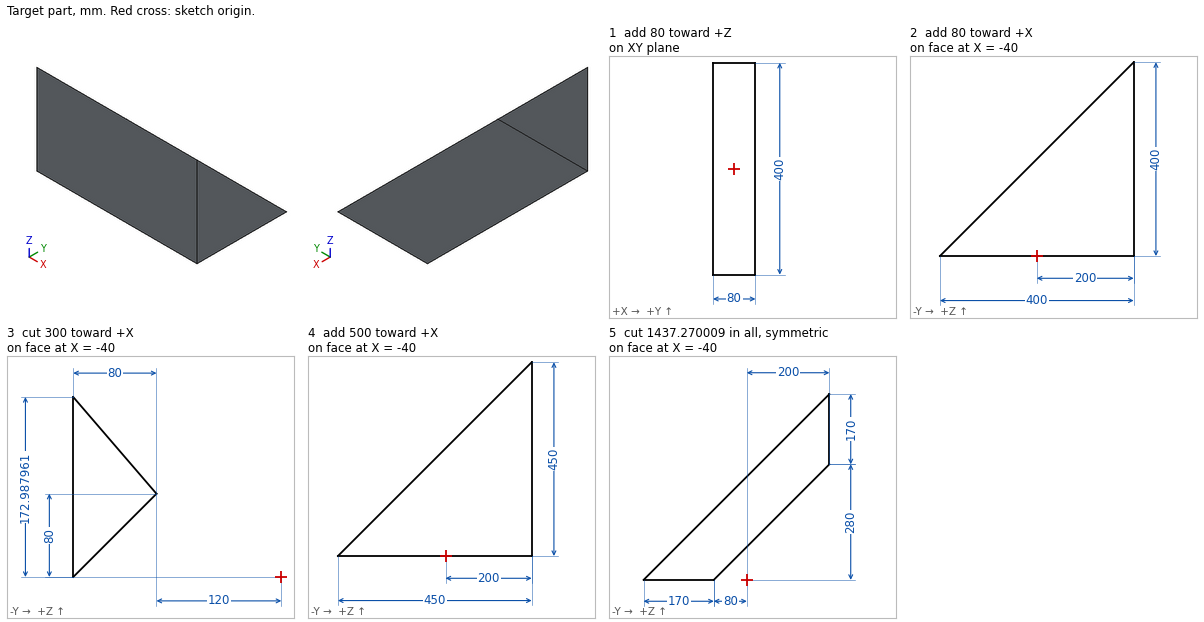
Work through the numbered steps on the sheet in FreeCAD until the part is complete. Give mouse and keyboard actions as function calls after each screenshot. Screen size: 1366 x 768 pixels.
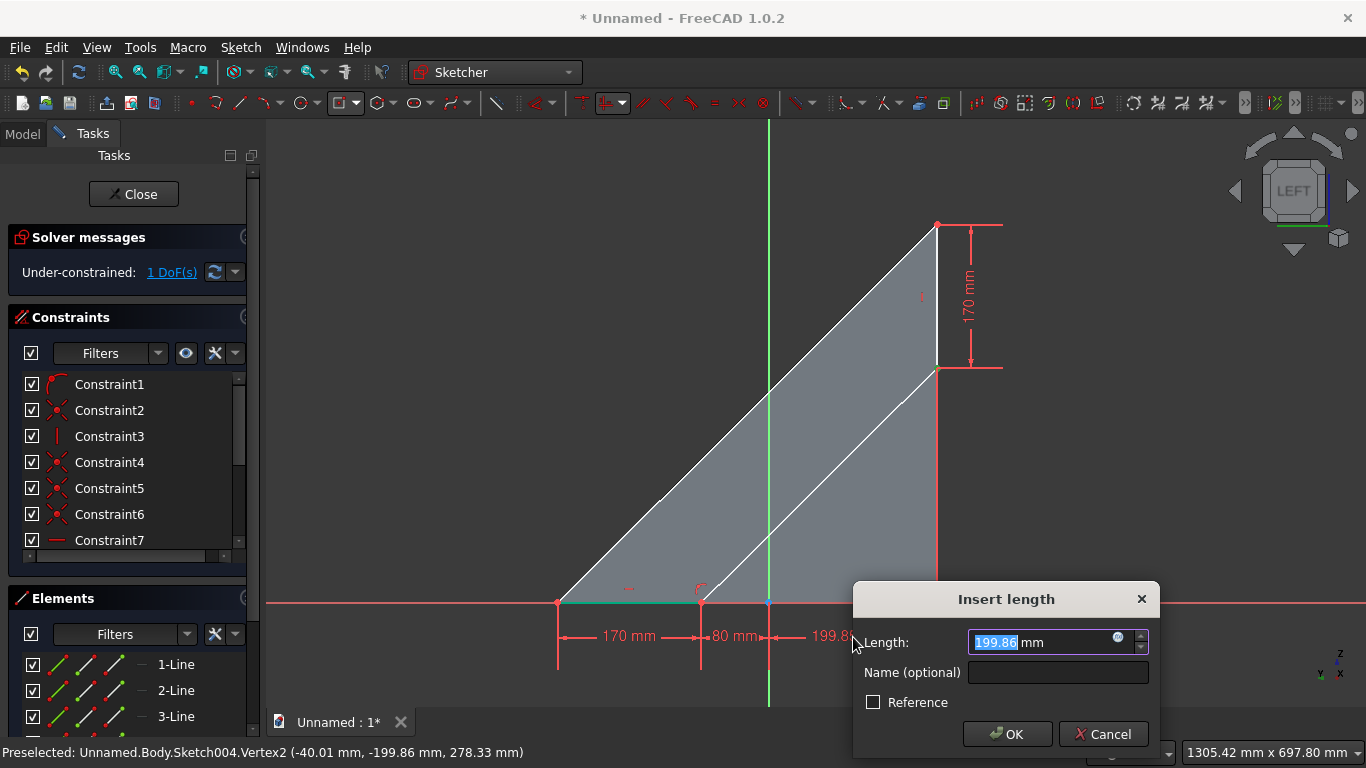
text(200)
key(Return)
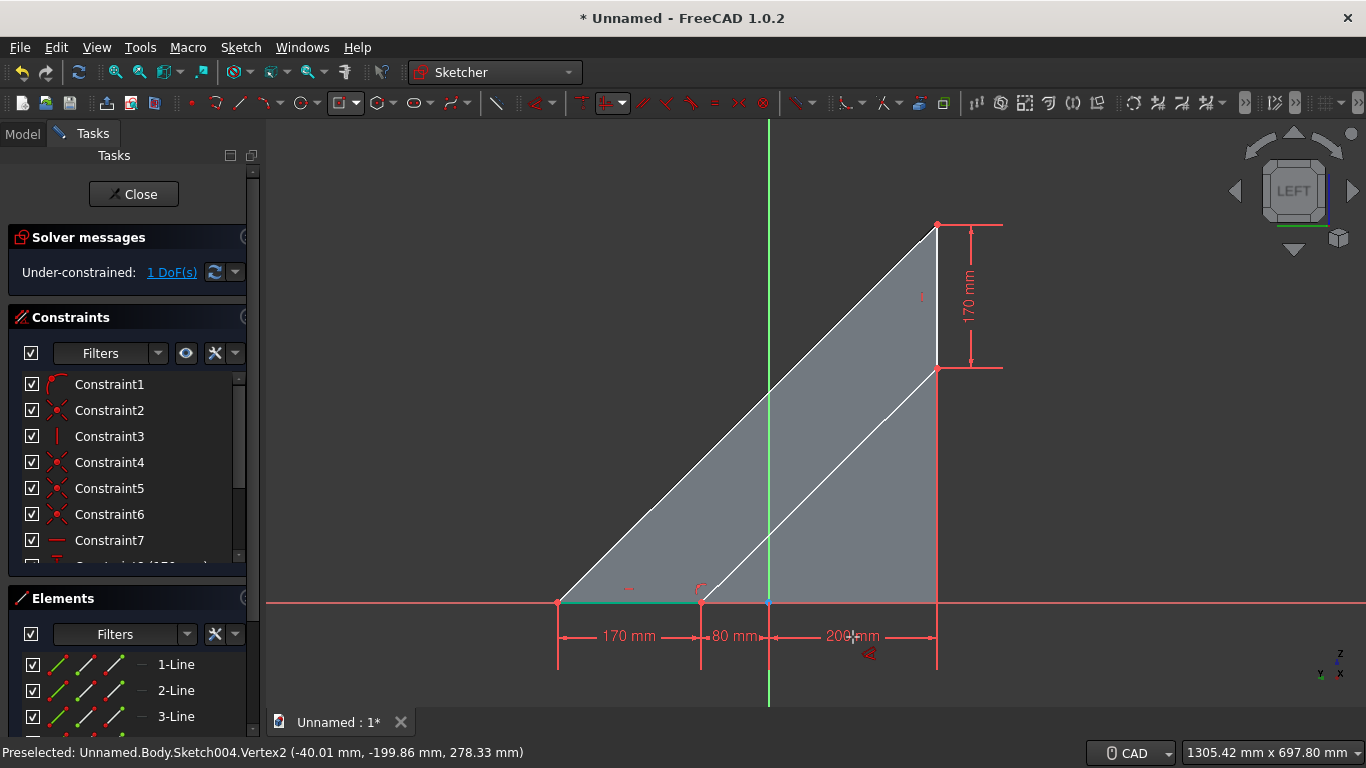
click(937, 368)
click(971, 485)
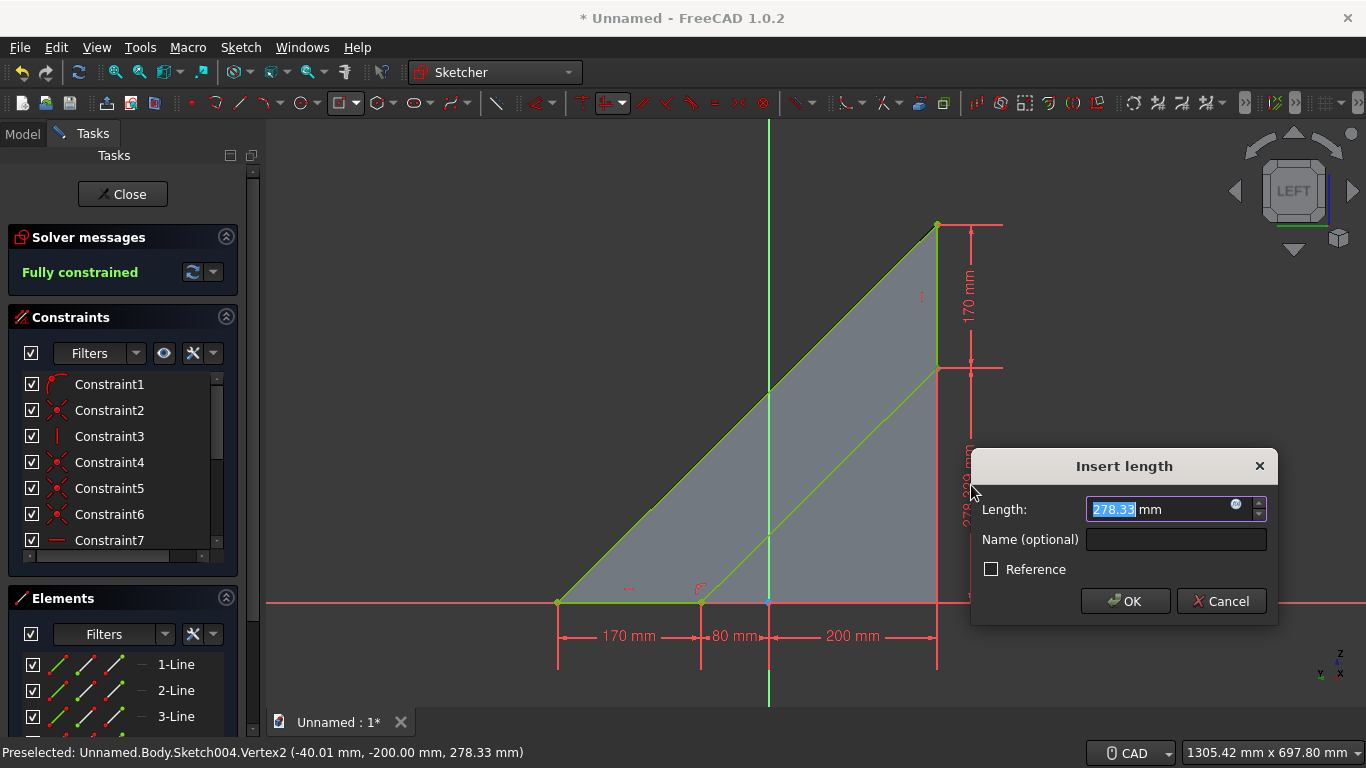
text(280)
key(Return)
key(Escape)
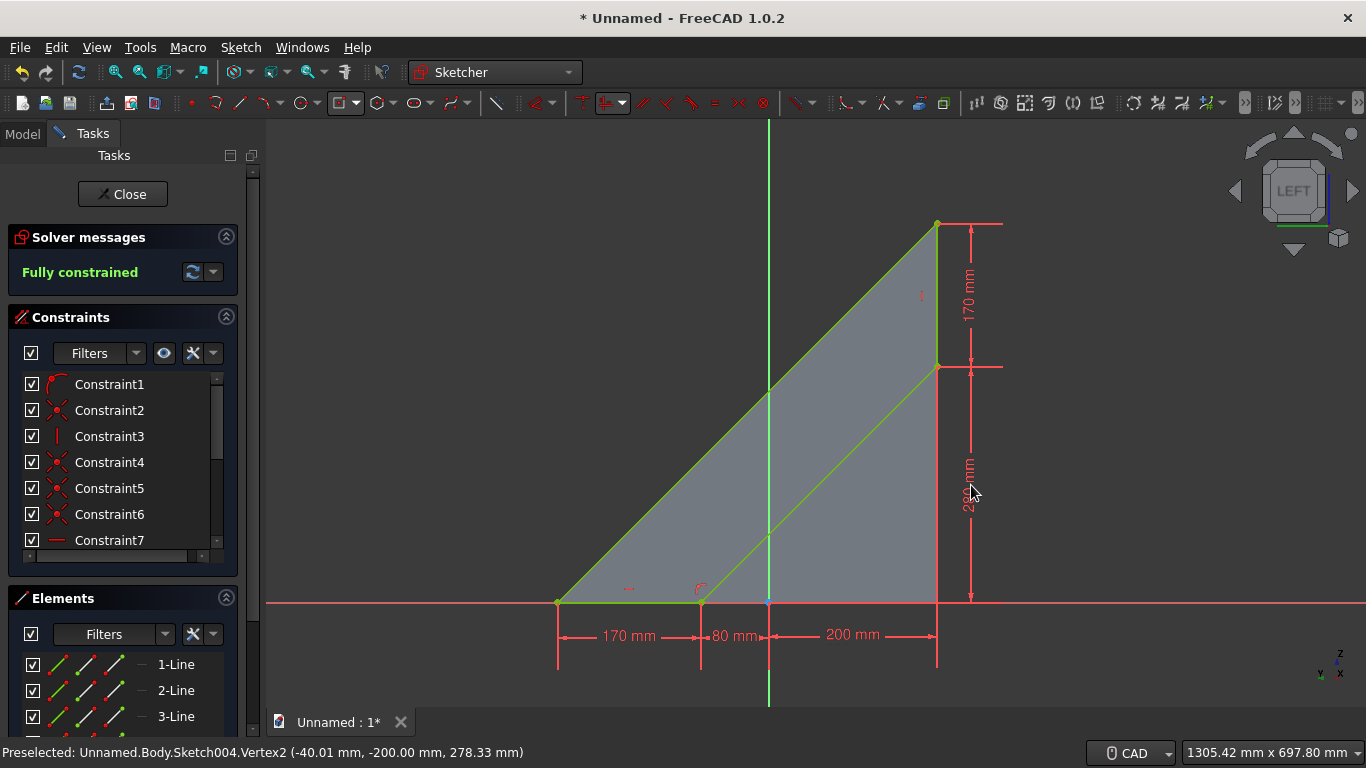
click(123, 194)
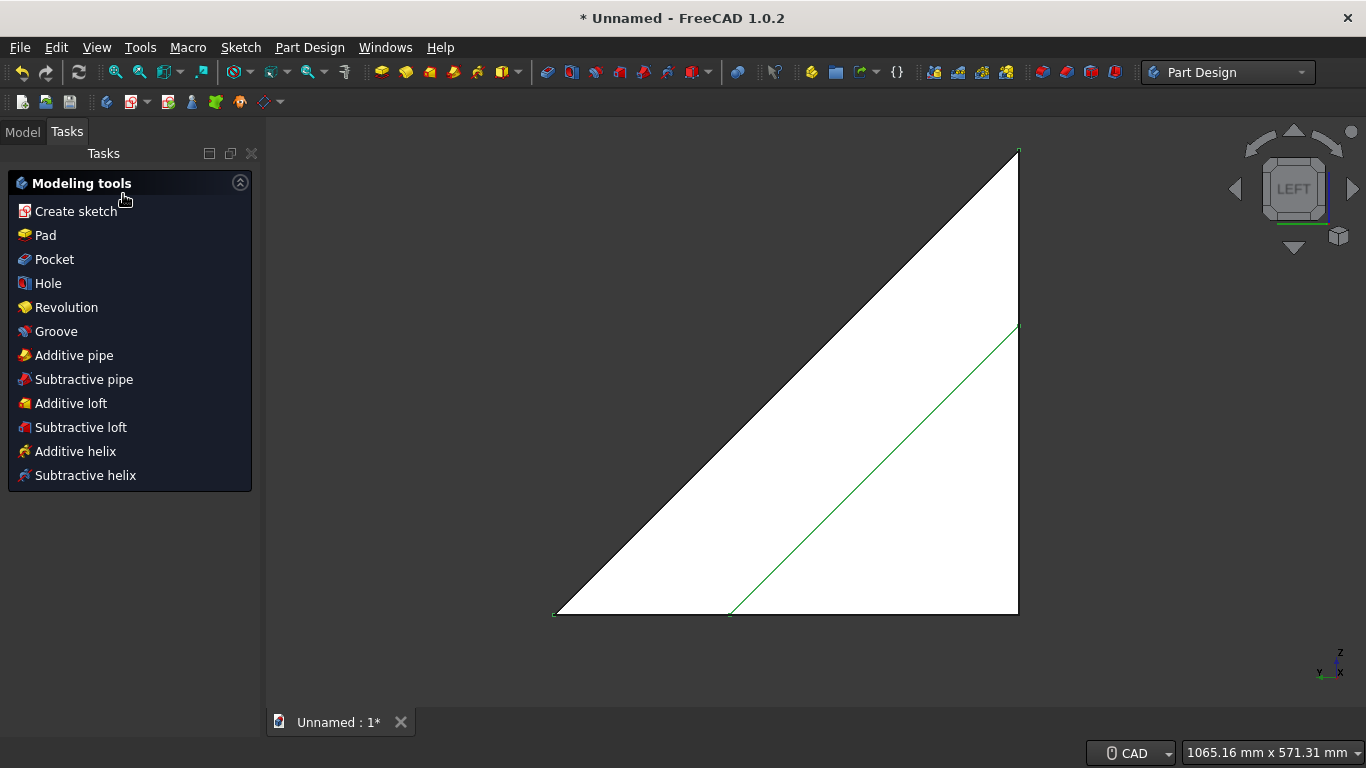
click(548, 72)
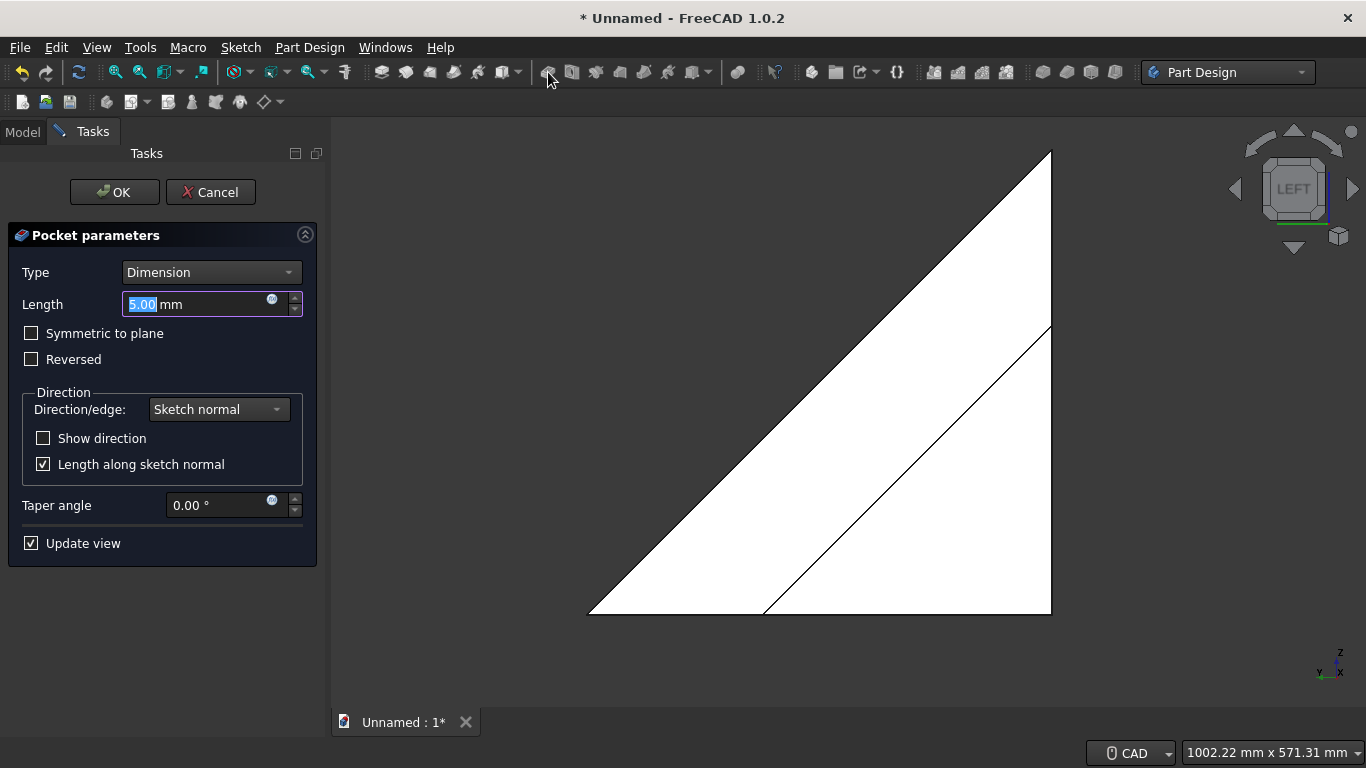
text(1437.270009)
key(Tab)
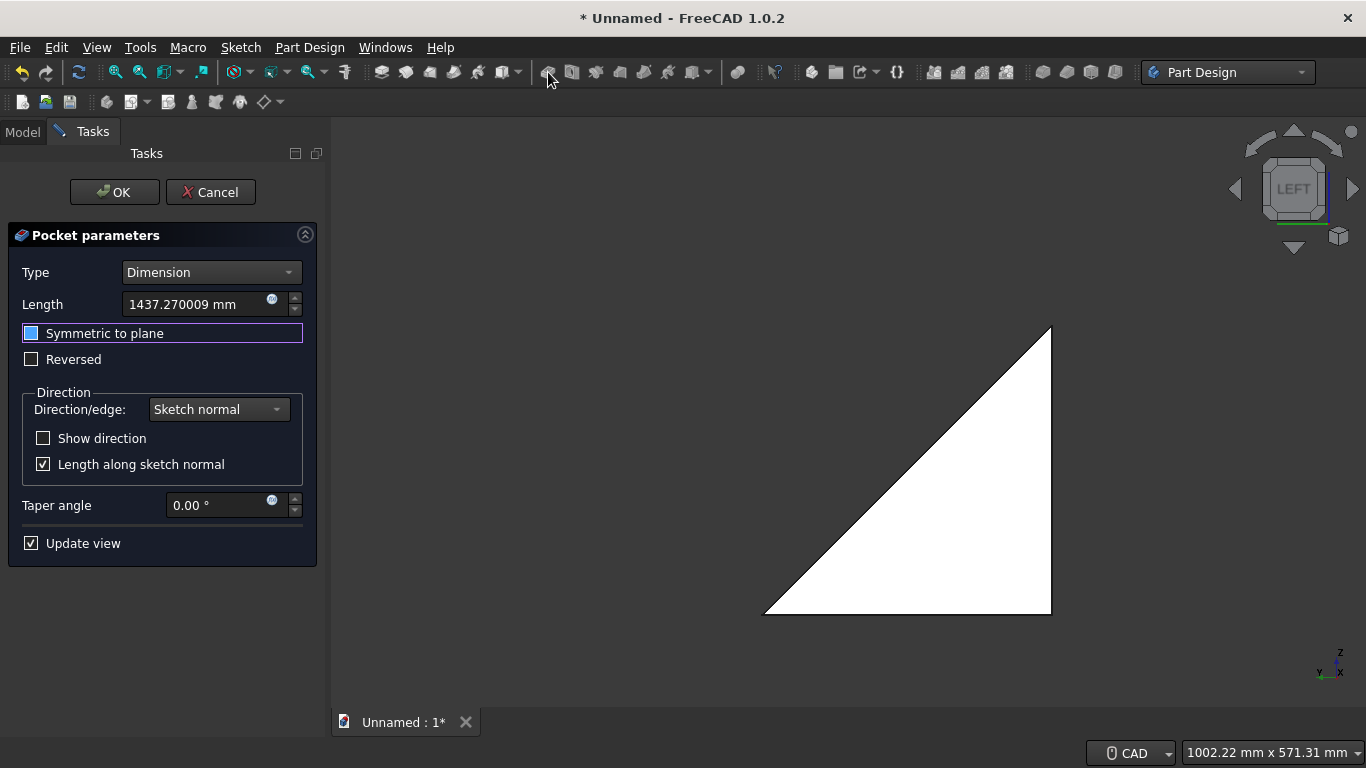
click(30, 333)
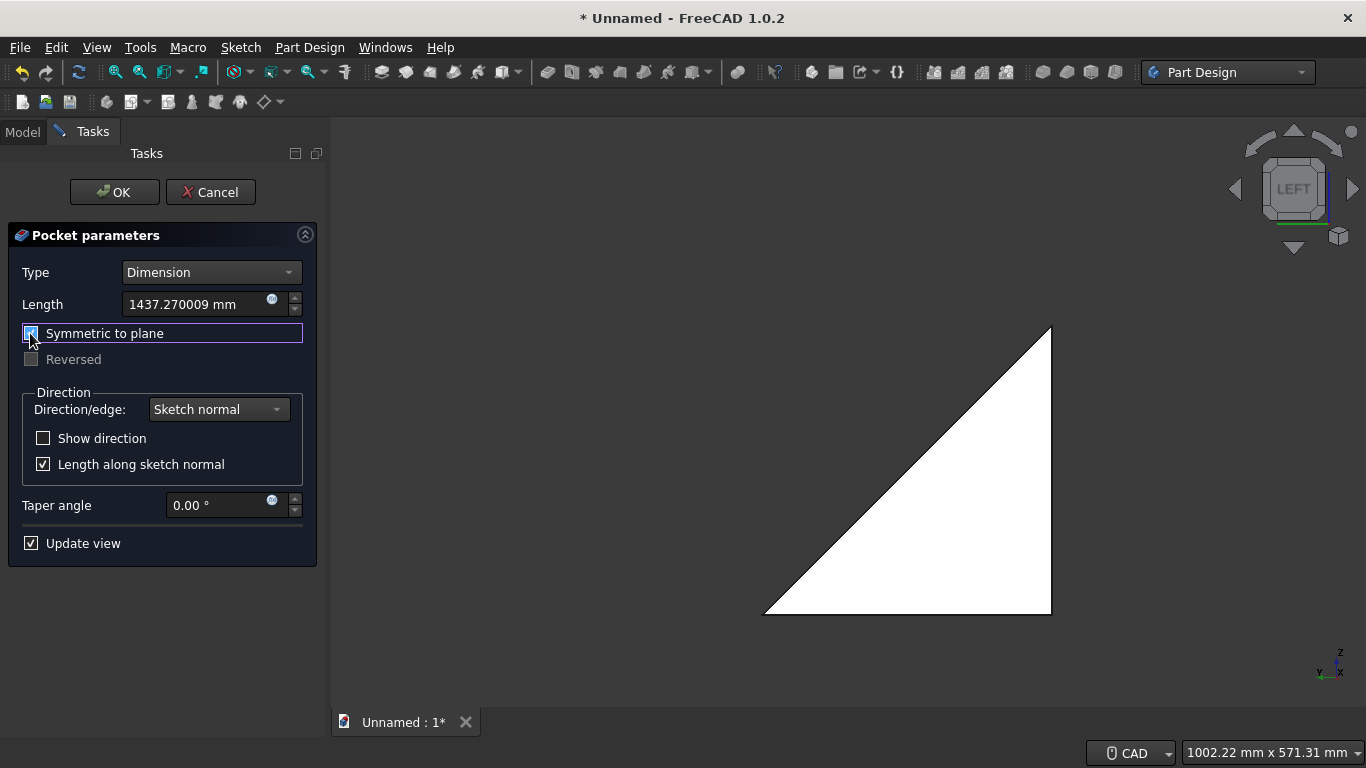
click(115, 192)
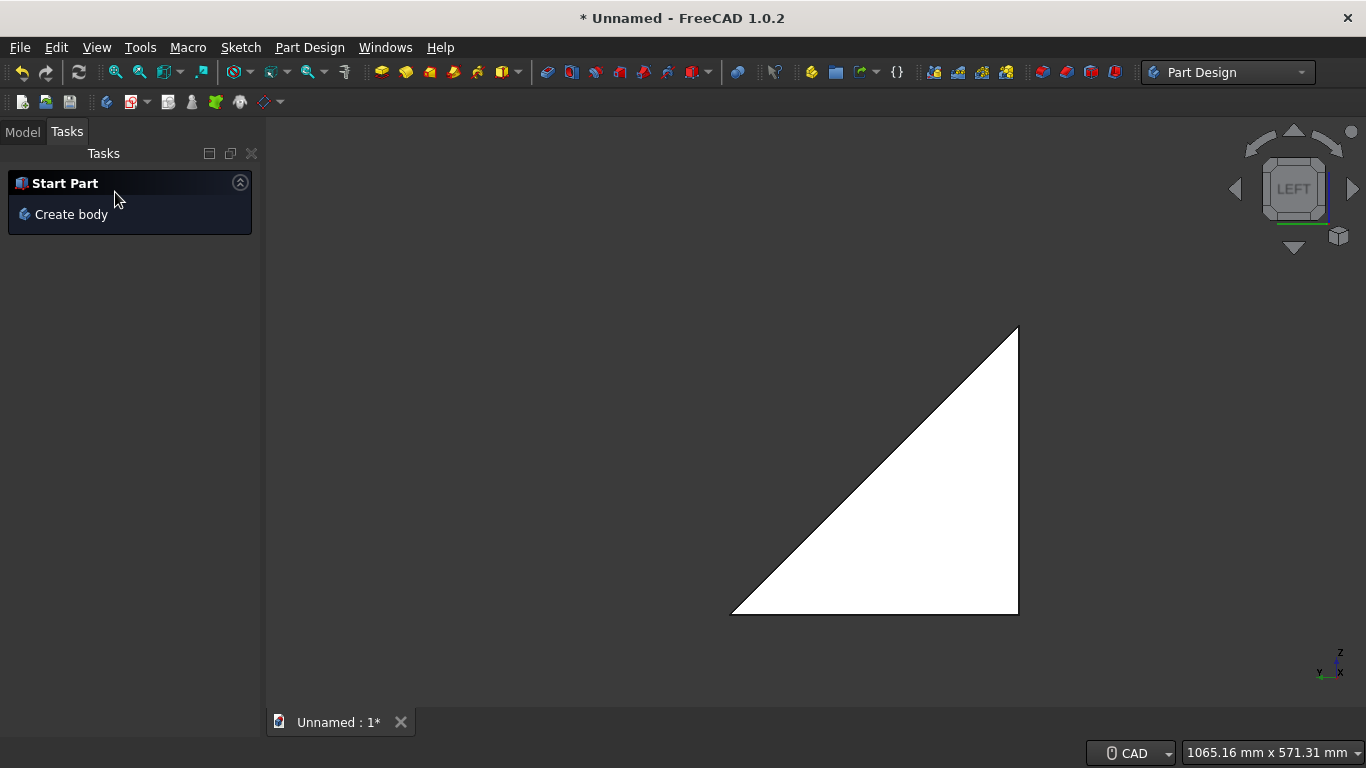
key(0)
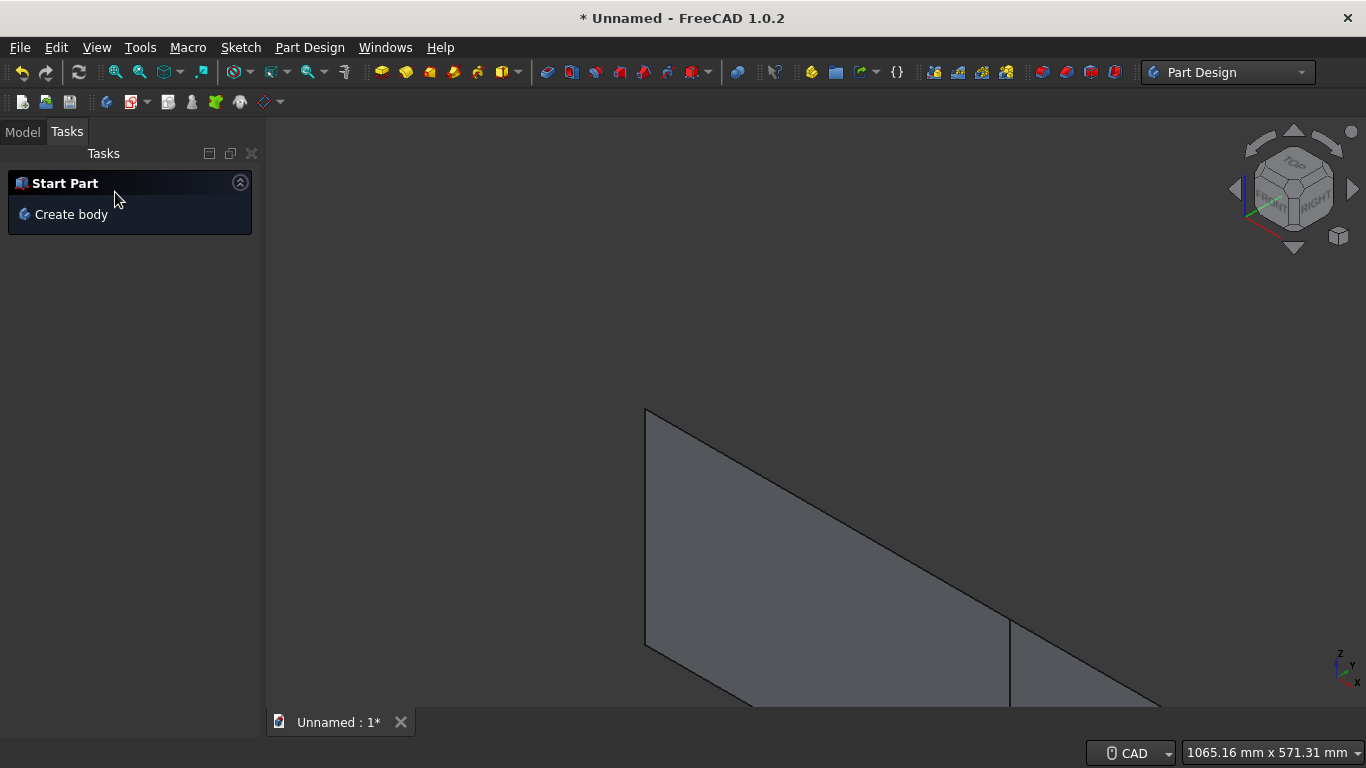
click(116, 72)